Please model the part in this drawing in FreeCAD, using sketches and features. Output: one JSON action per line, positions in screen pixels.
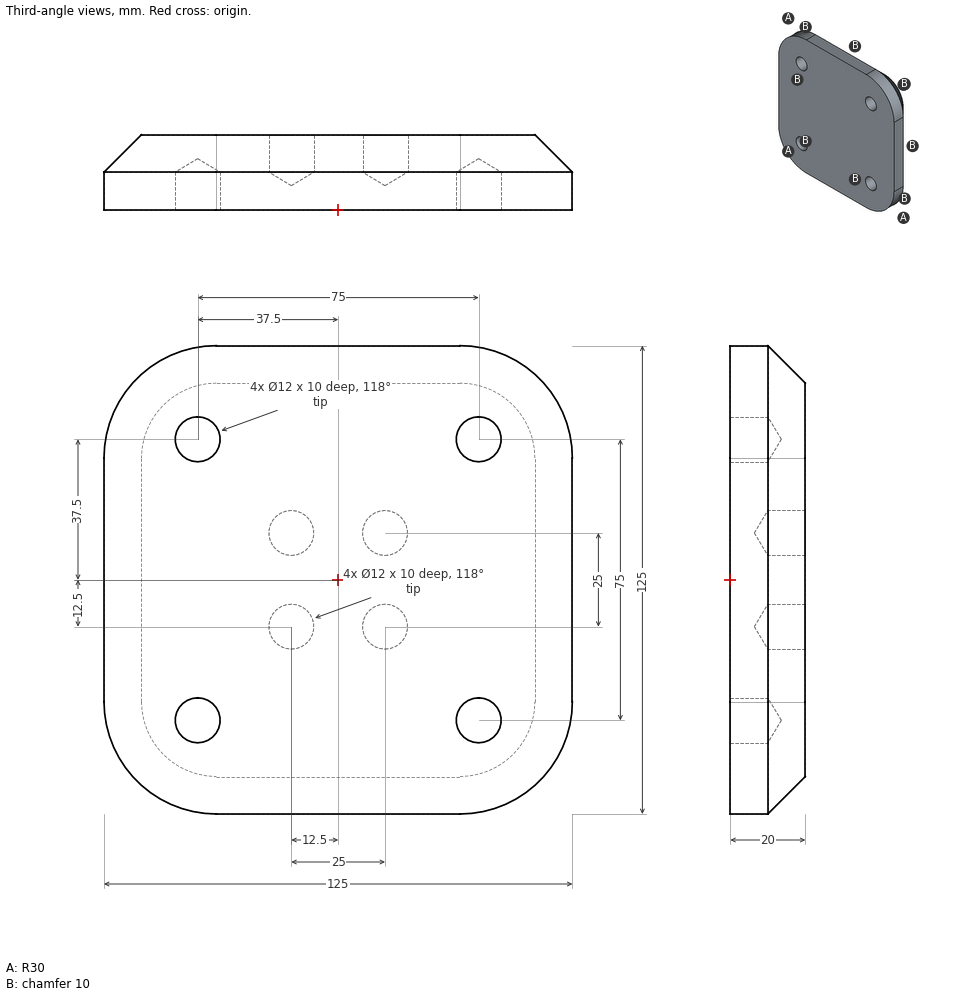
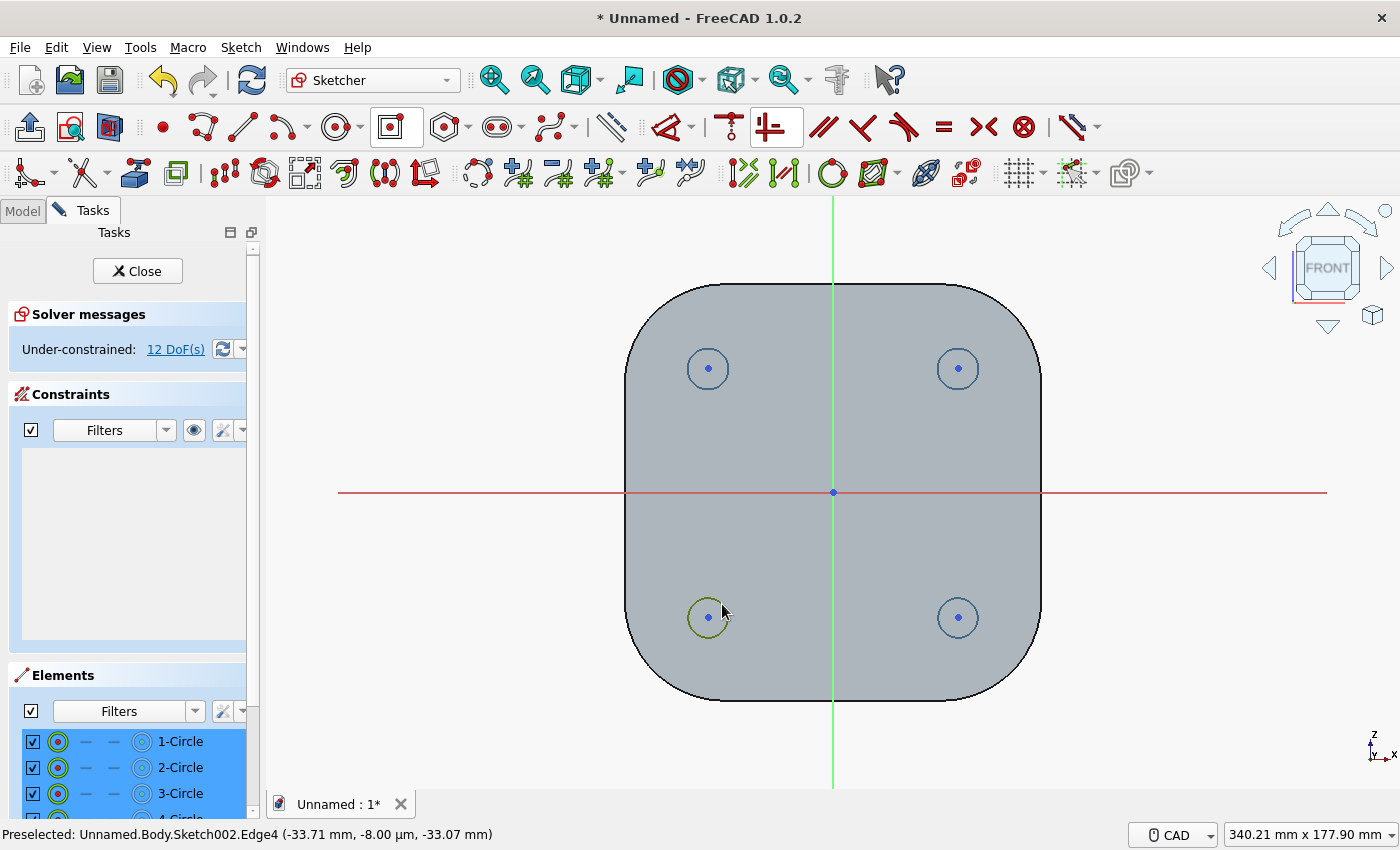
{"action": "key", "text": "e"}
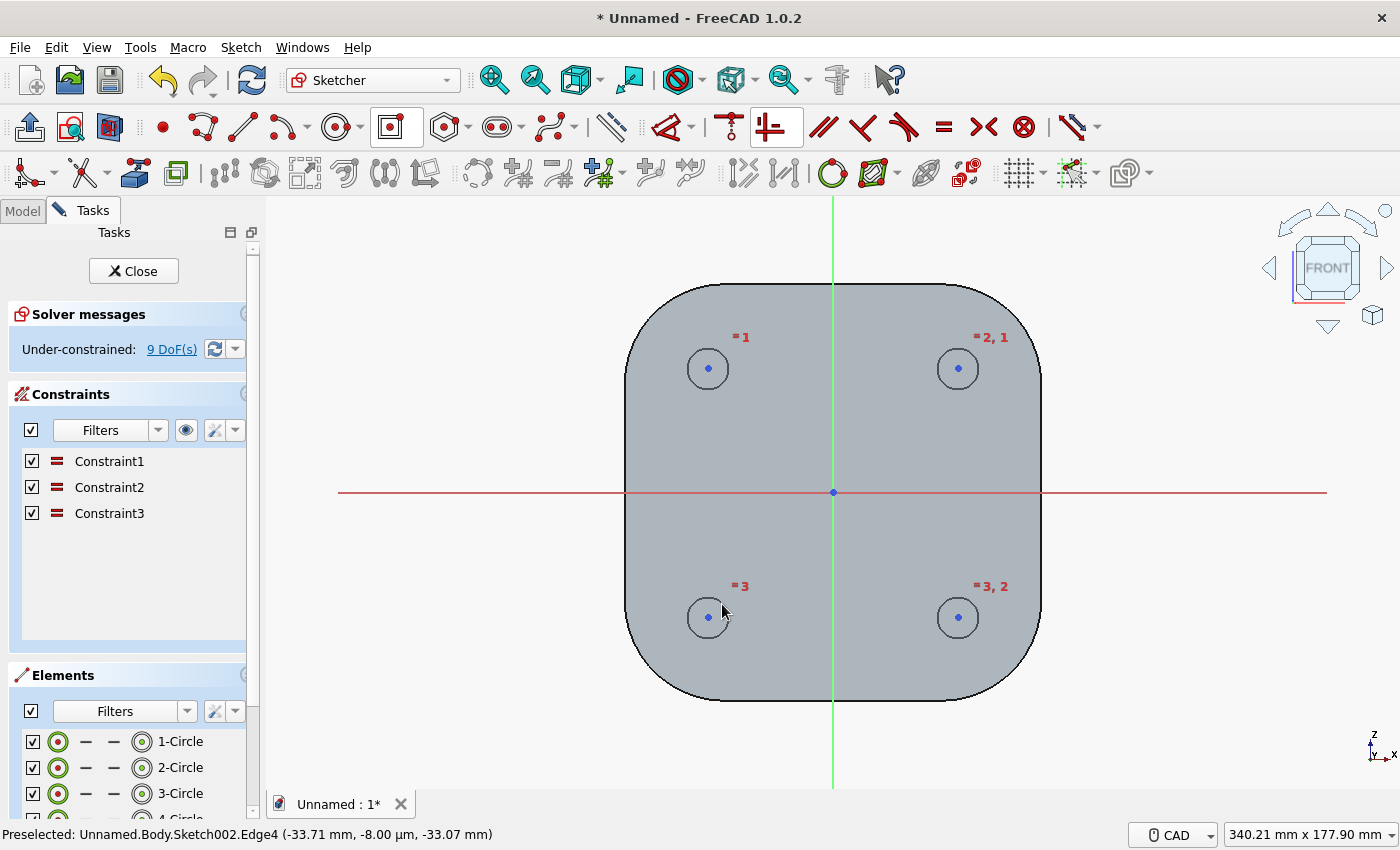
{"action": "left_click", "coordinate": [708, 369]}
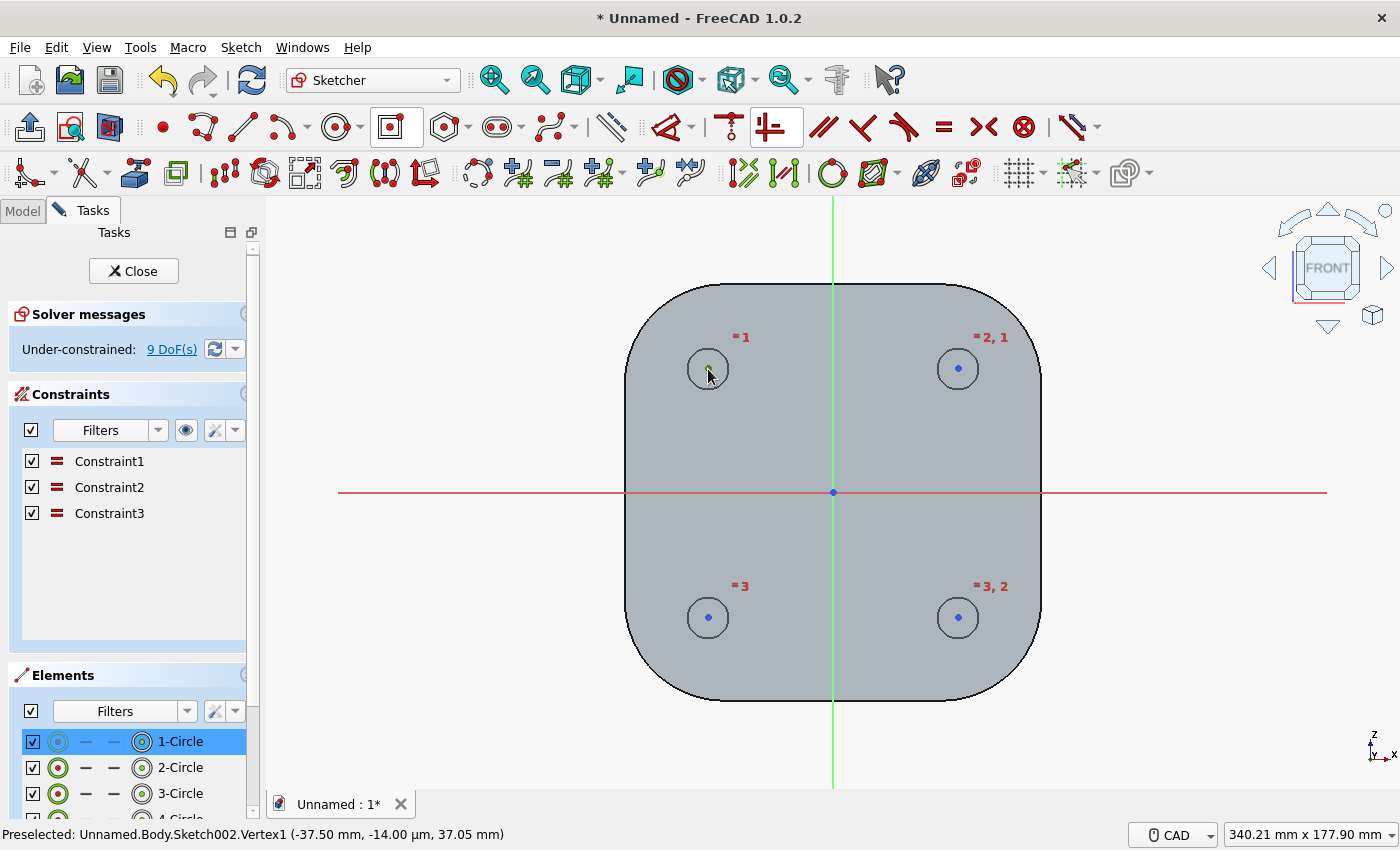
{"action": "left_click", "coordinate": [958, 369]}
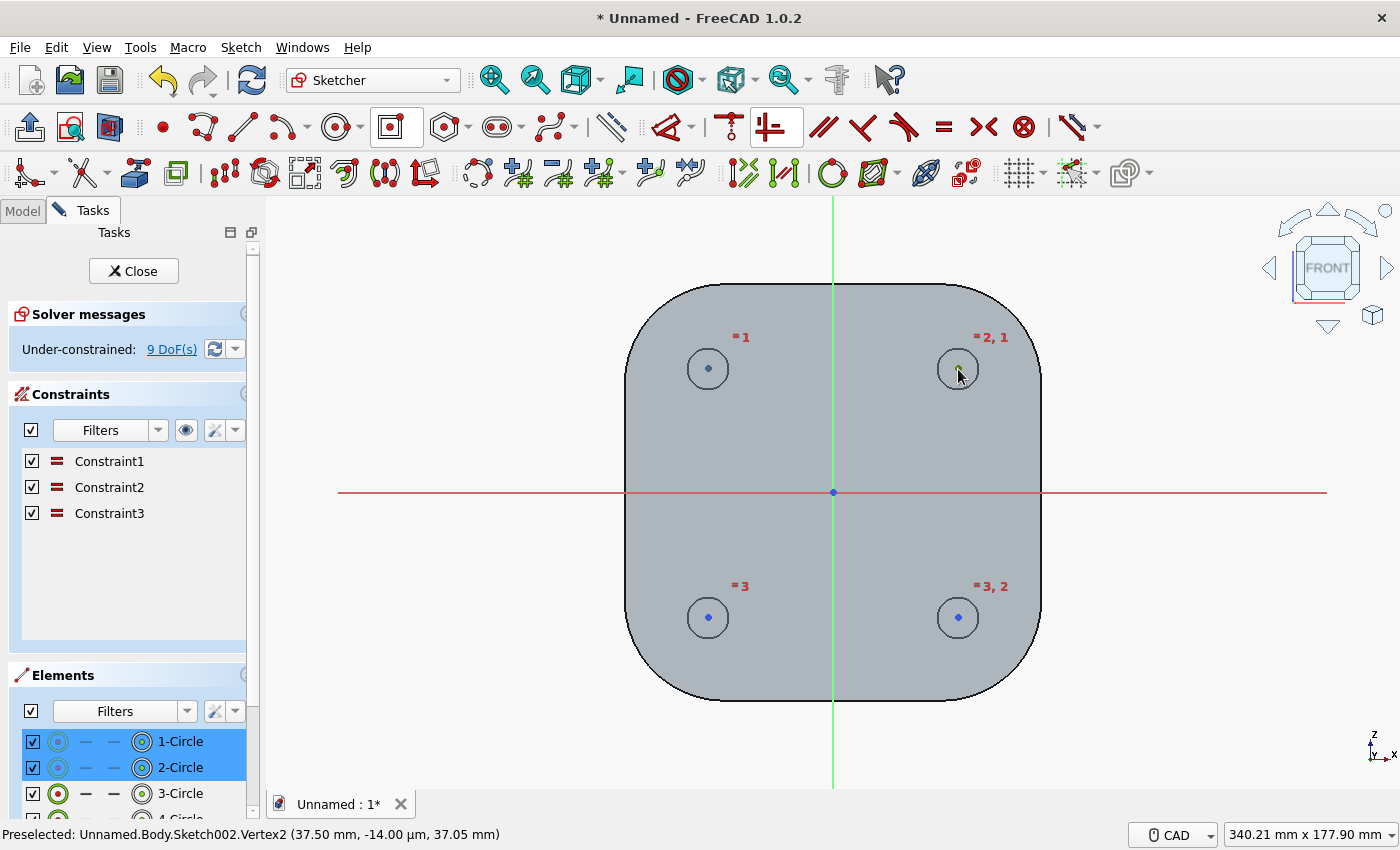
{"action": "key", "text": "h"}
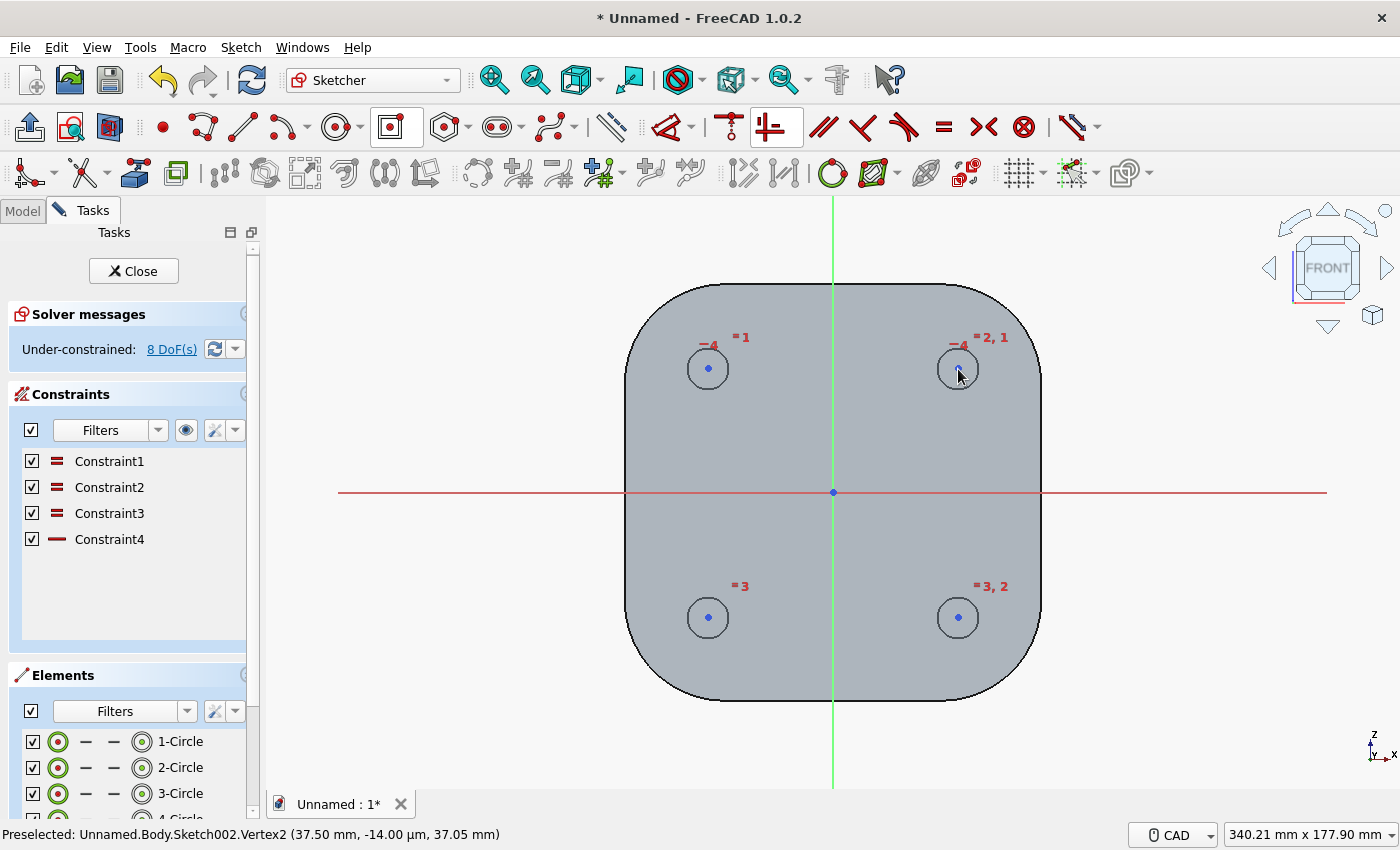
{"action": "left_click", "coordinate": [958, 369]}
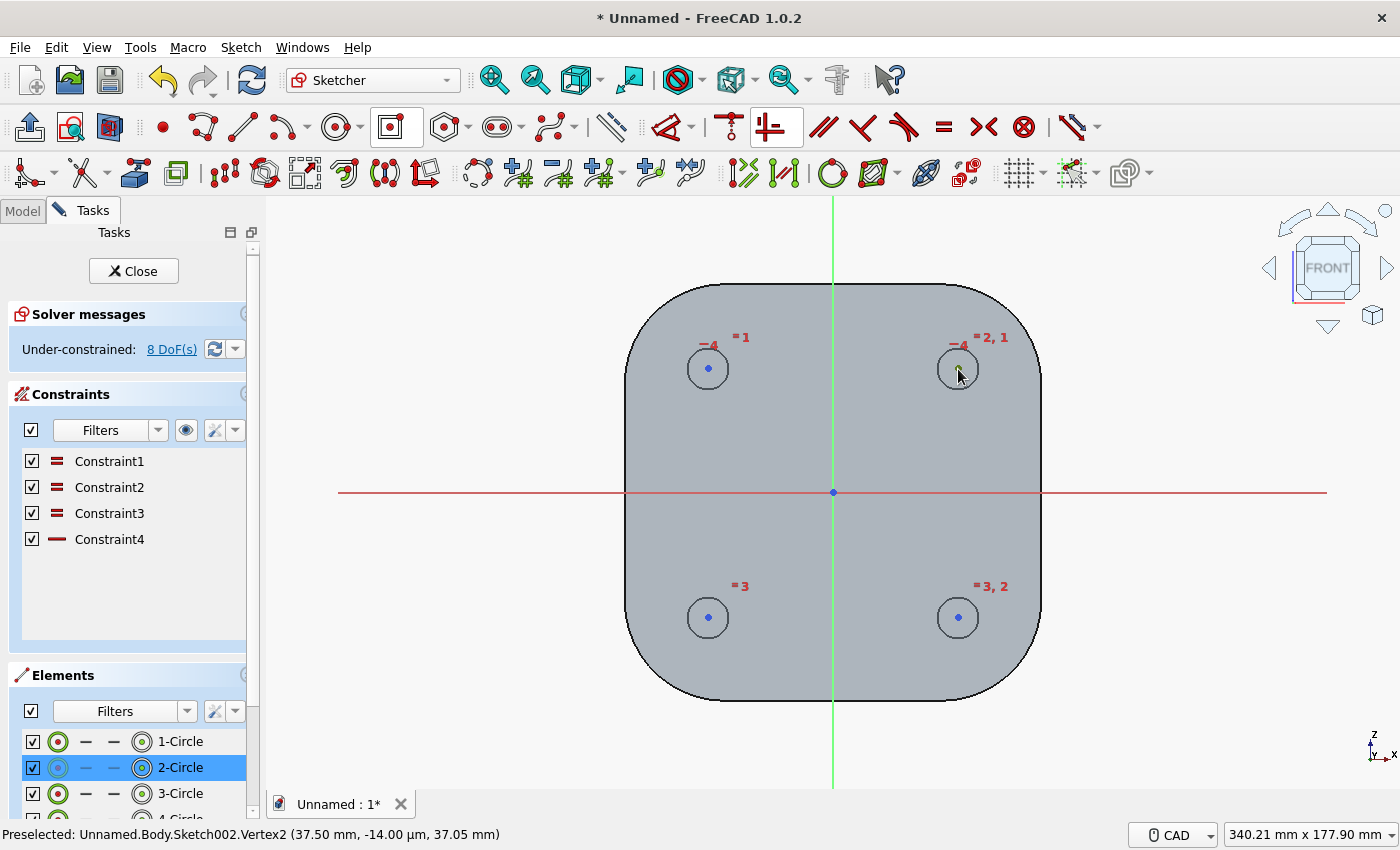
{"action": "left_click", "coordinate": [958, 618]}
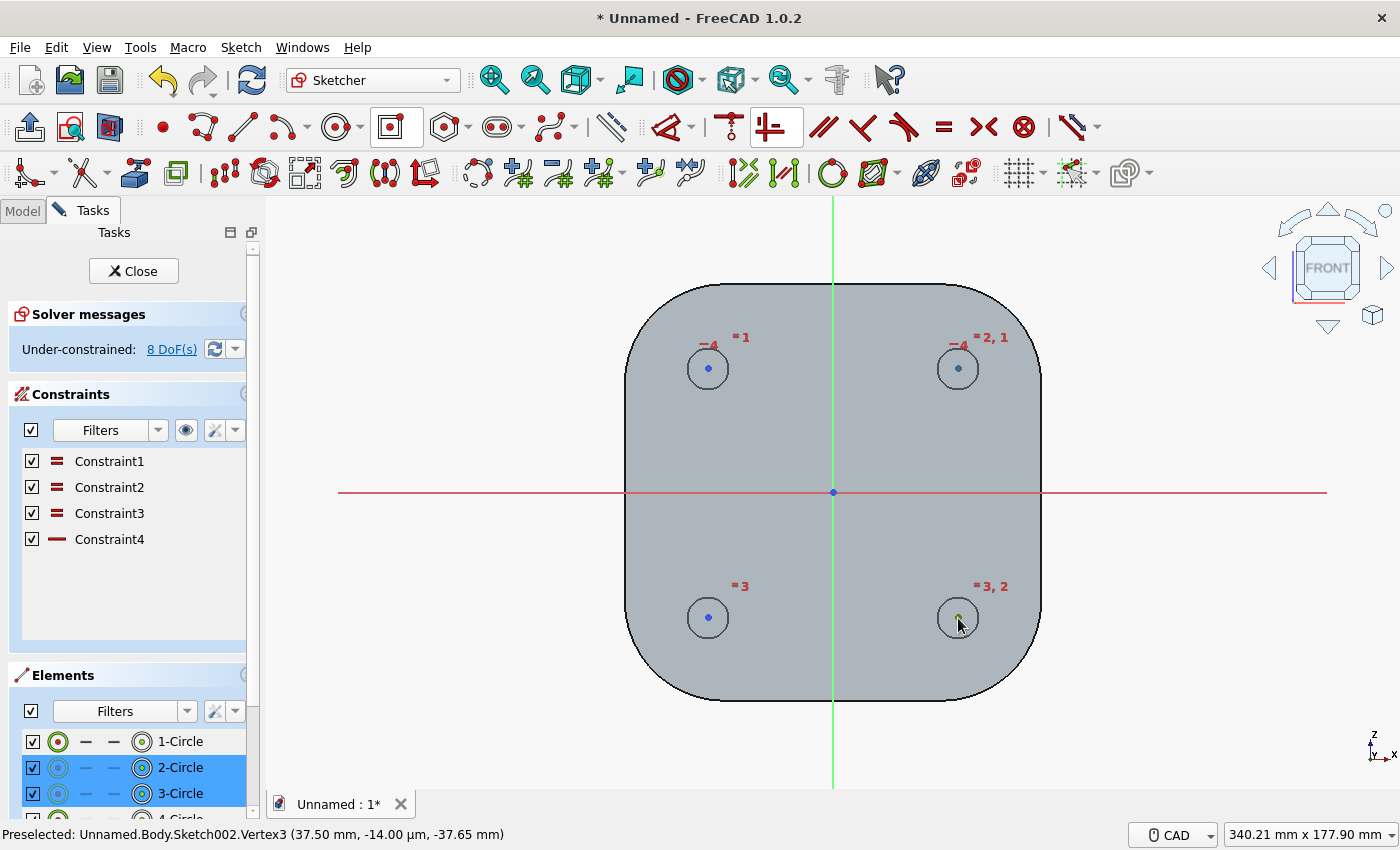
{"action": "key", "text": "v"}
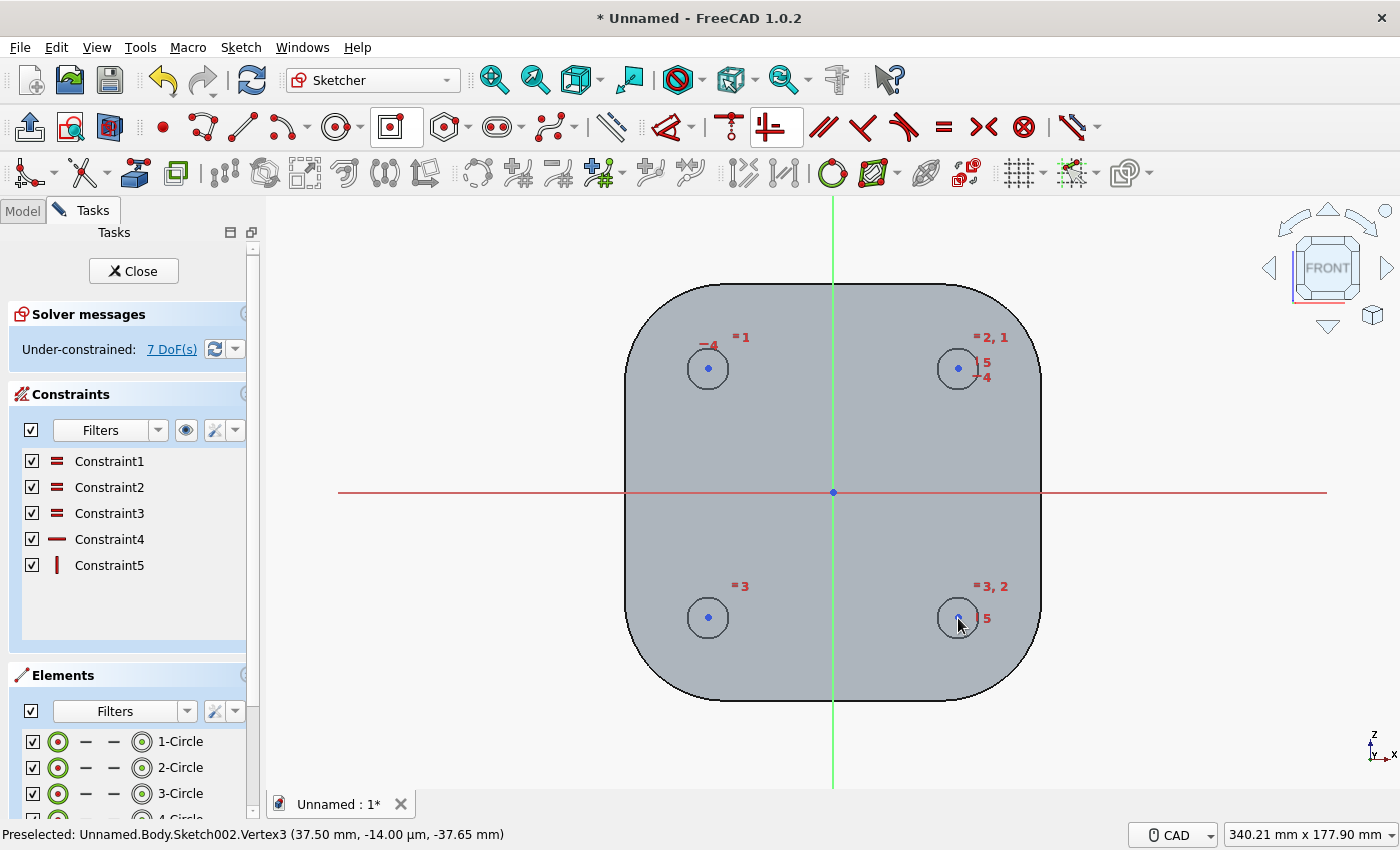
{"action": "left_click", "coordinate": [708, 369]}